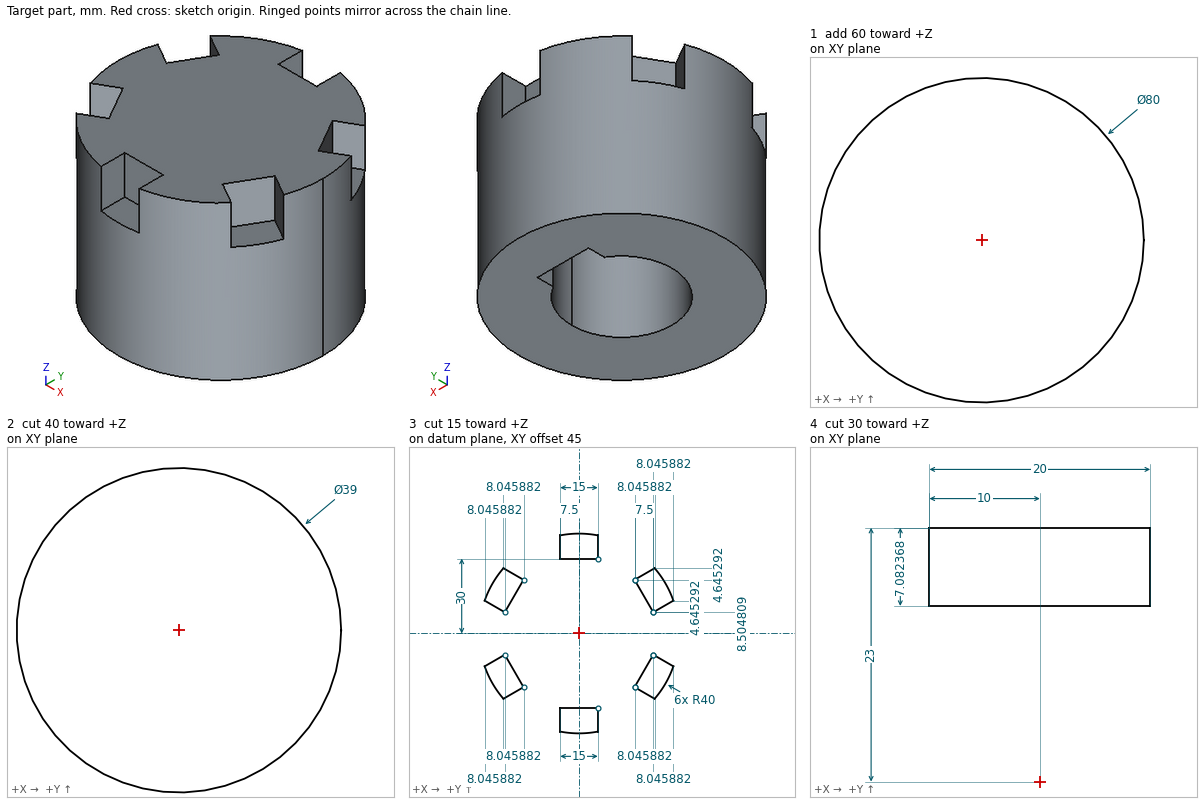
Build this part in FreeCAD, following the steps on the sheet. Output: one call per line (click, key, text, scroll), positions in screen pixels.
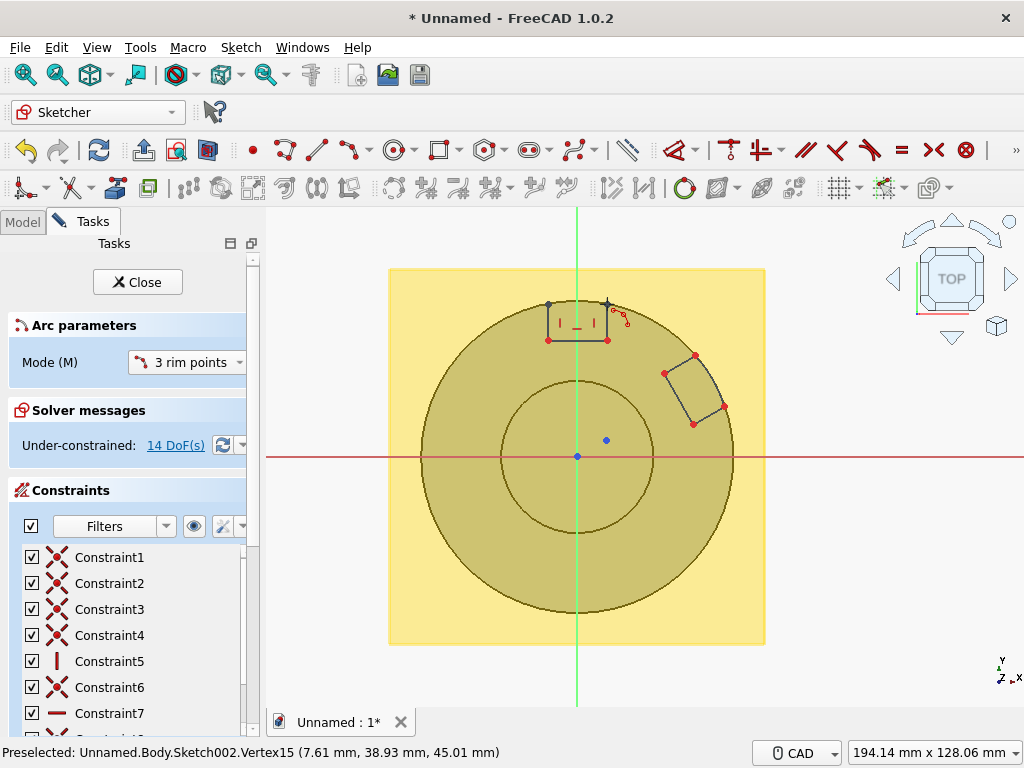
click(607, 305)
click(548, 305)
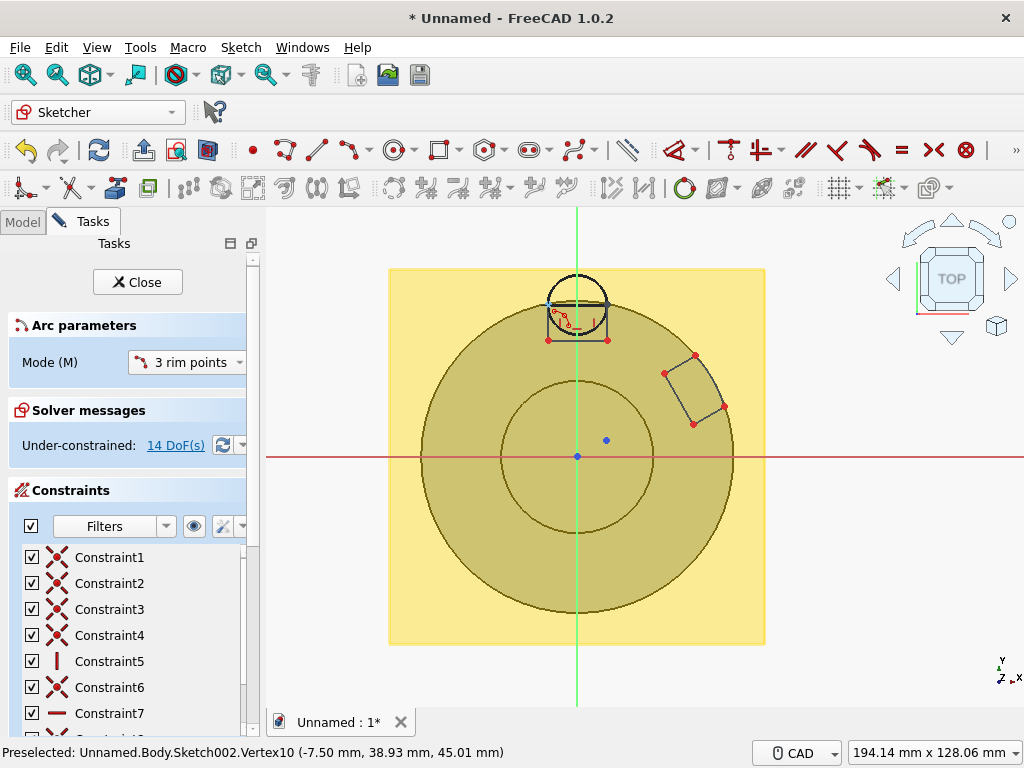
scroll(583, 301, up, 9)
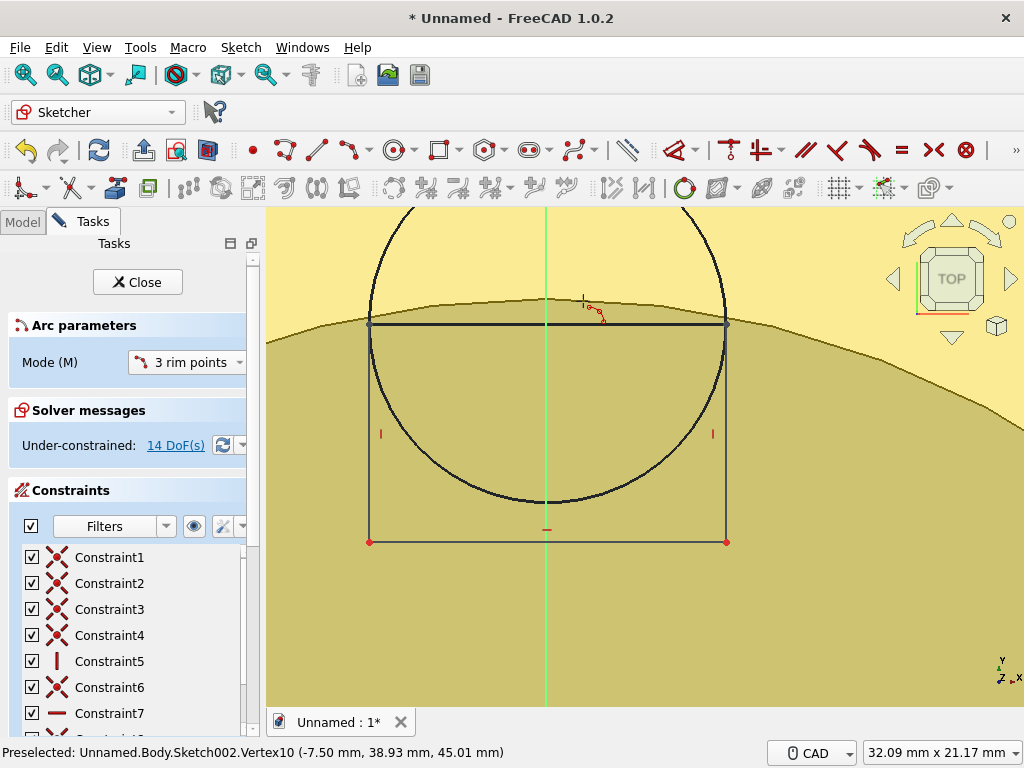
click(582, 300)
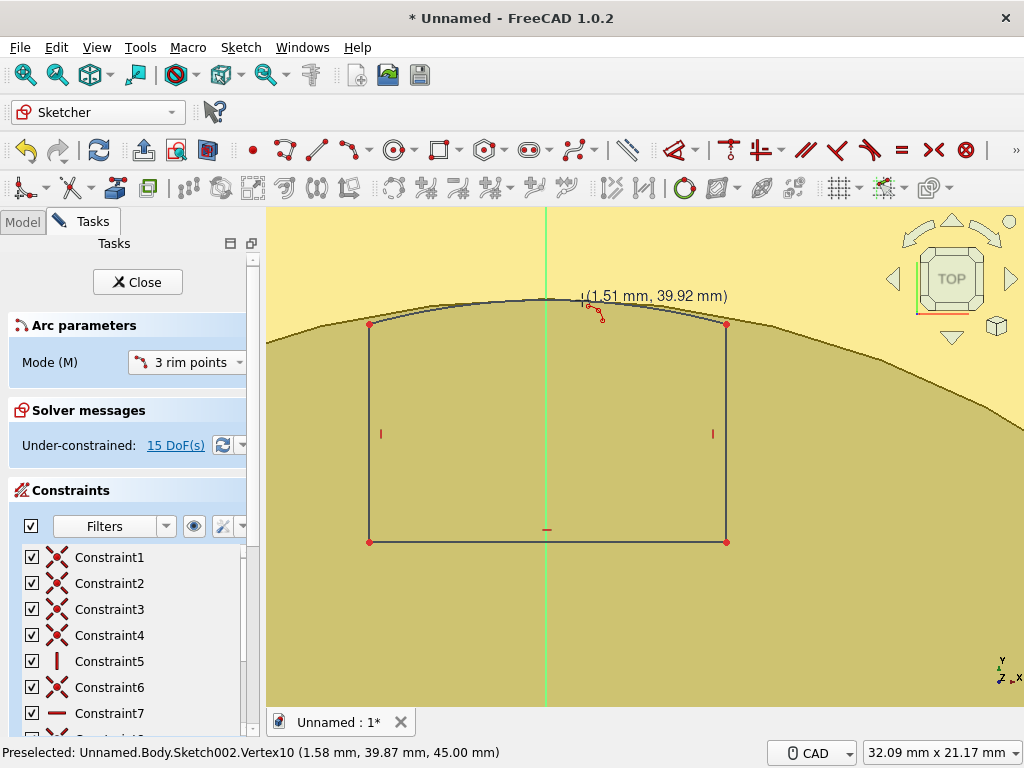
click(286, 150)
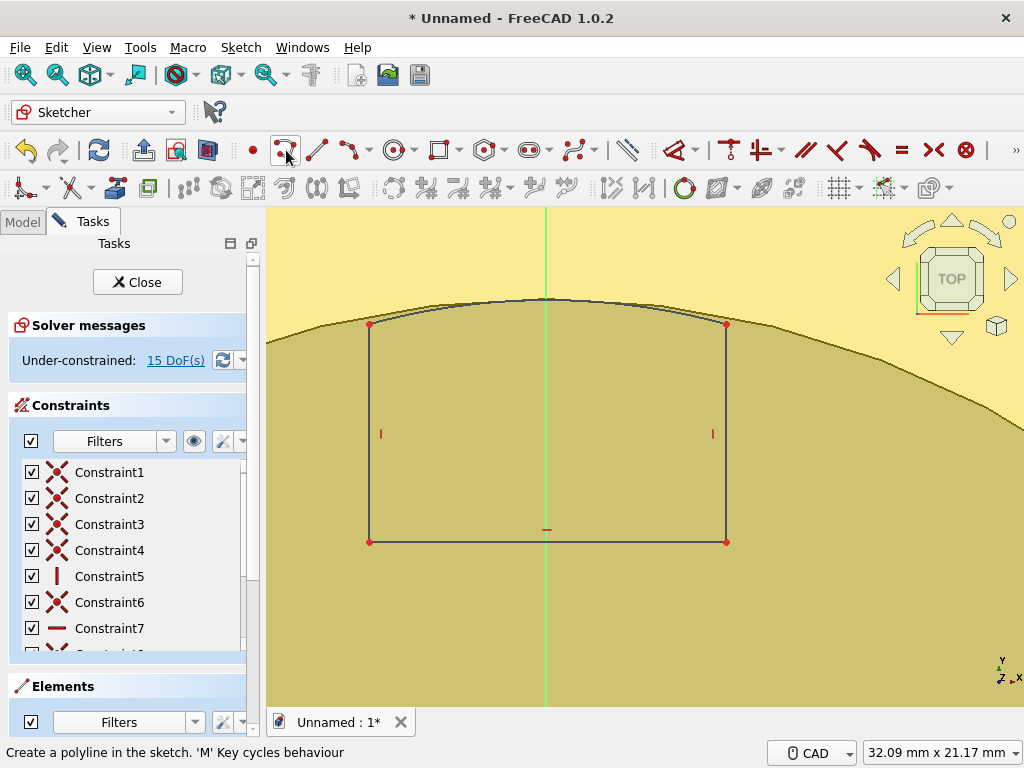
scroll(582, 301, down, 9)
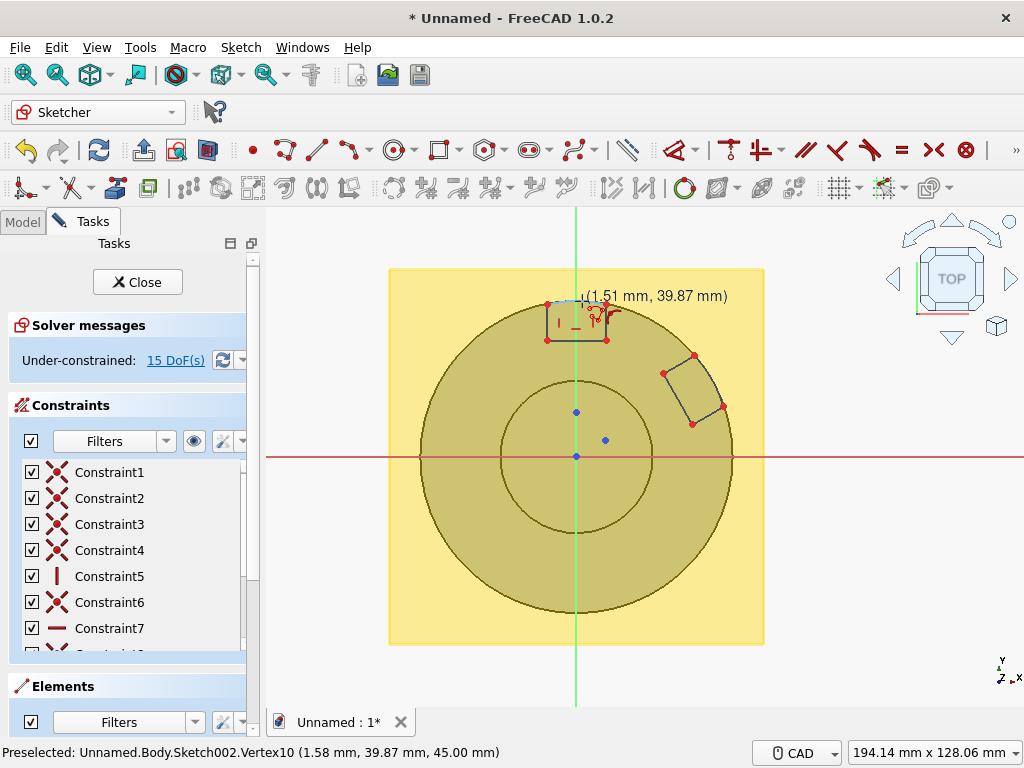
click(724, 508)
click(693, 490)
click(663, 541)
click(695, 559)
right_click(695, 559)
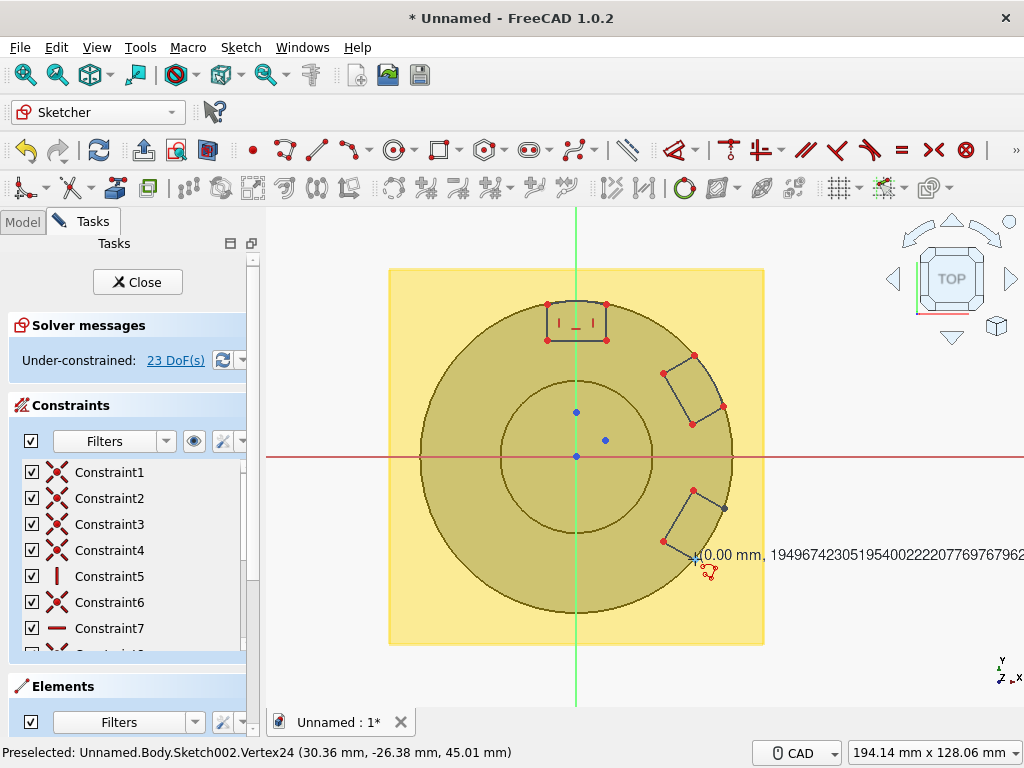
click(350, 150)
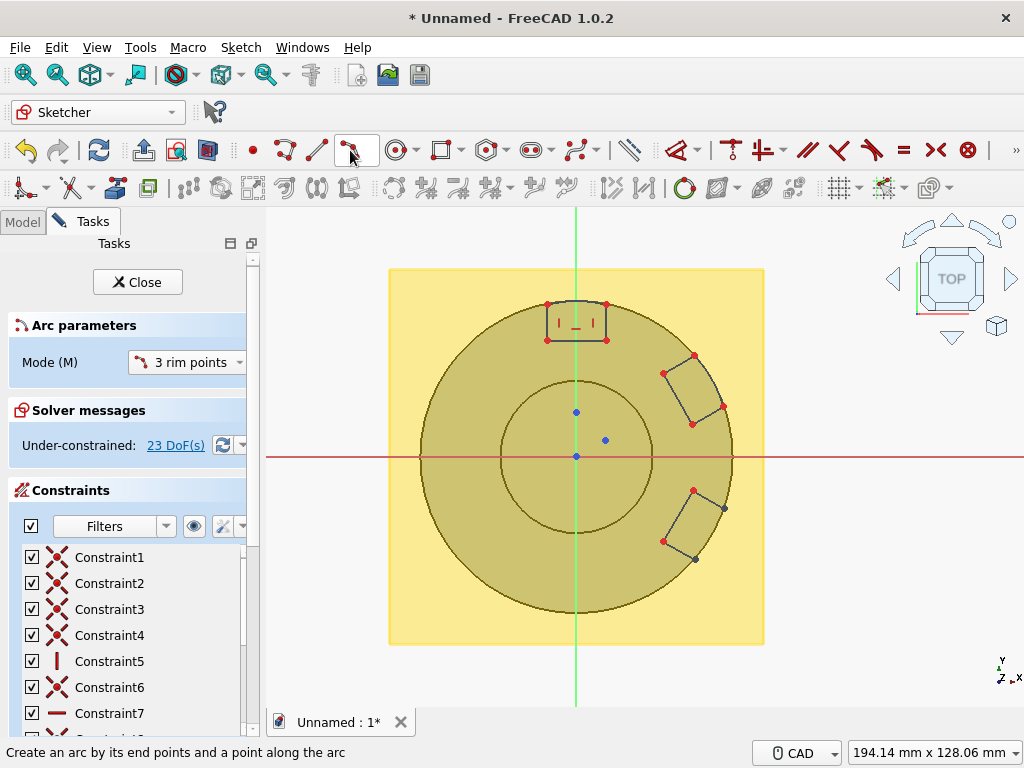
click(695, 560)
click(724, 509)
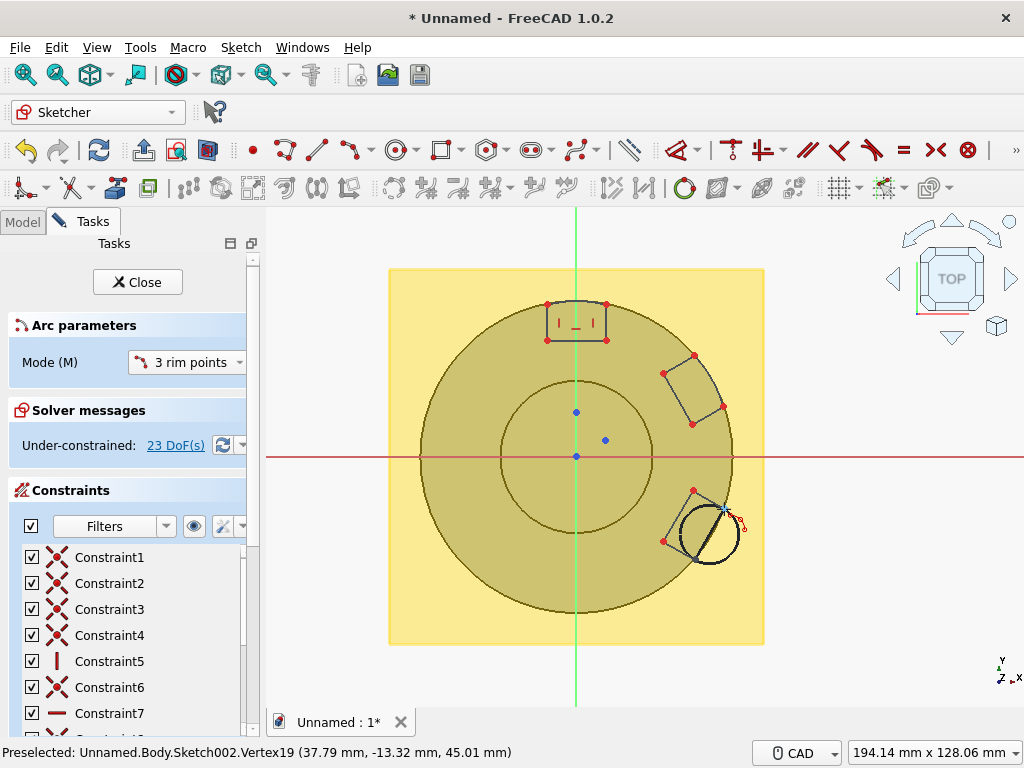
scroll(712, 535, up, 9)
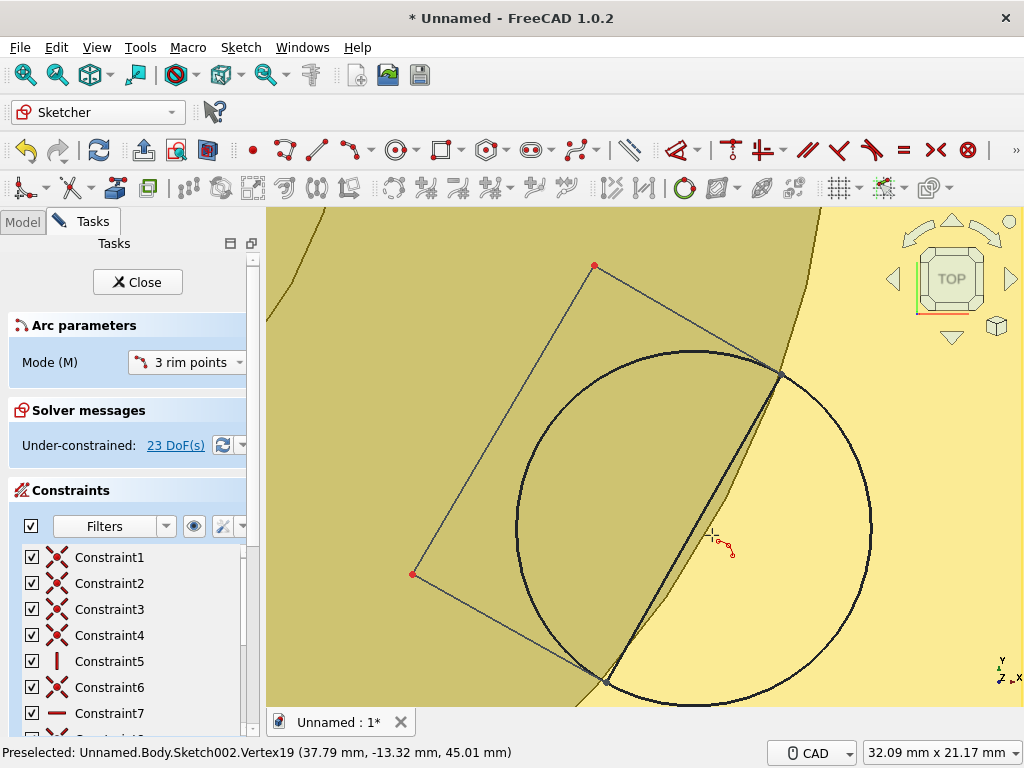
click(707, 532)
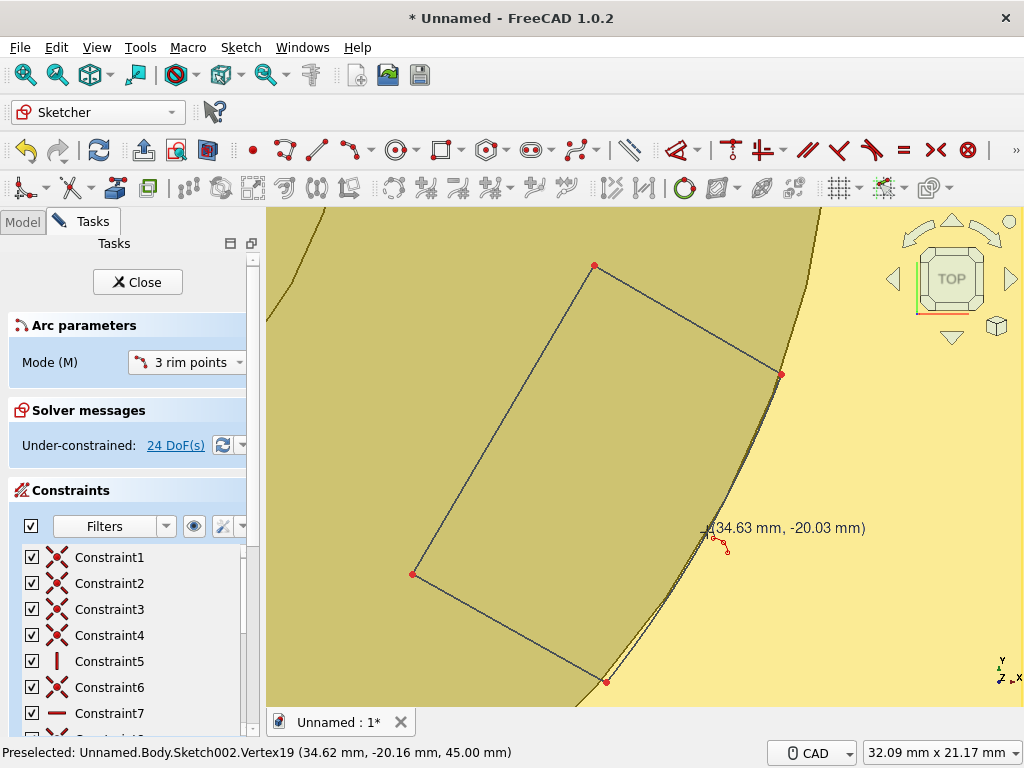
click(286, 150)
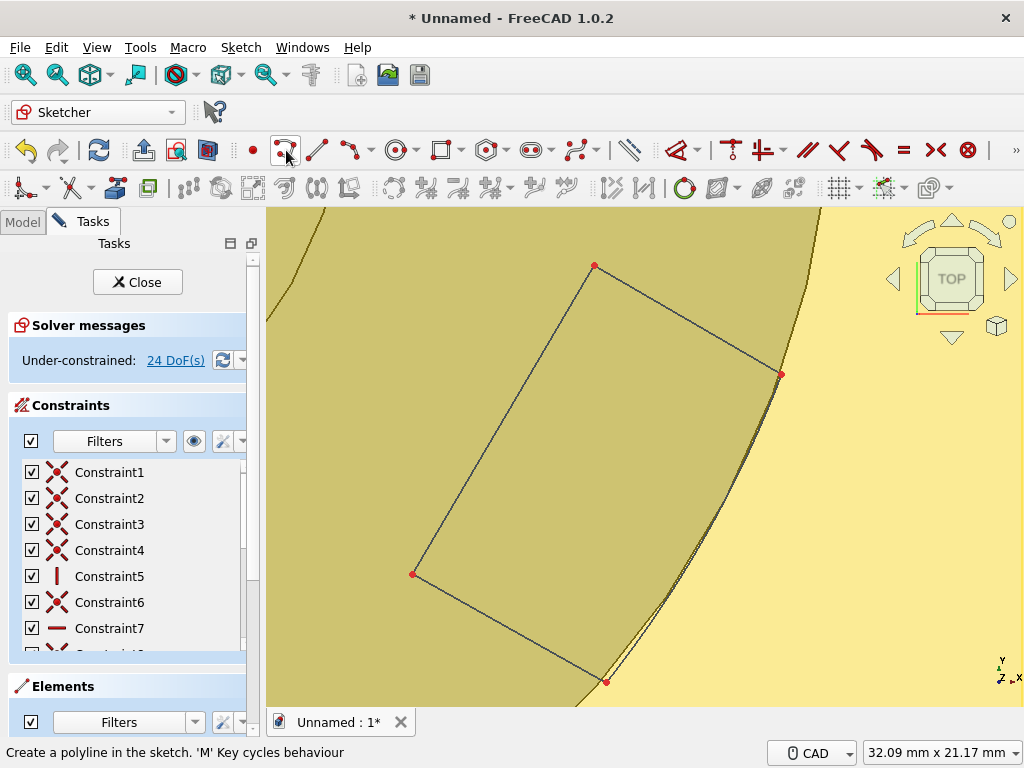
scroll(713, 536, down, 9)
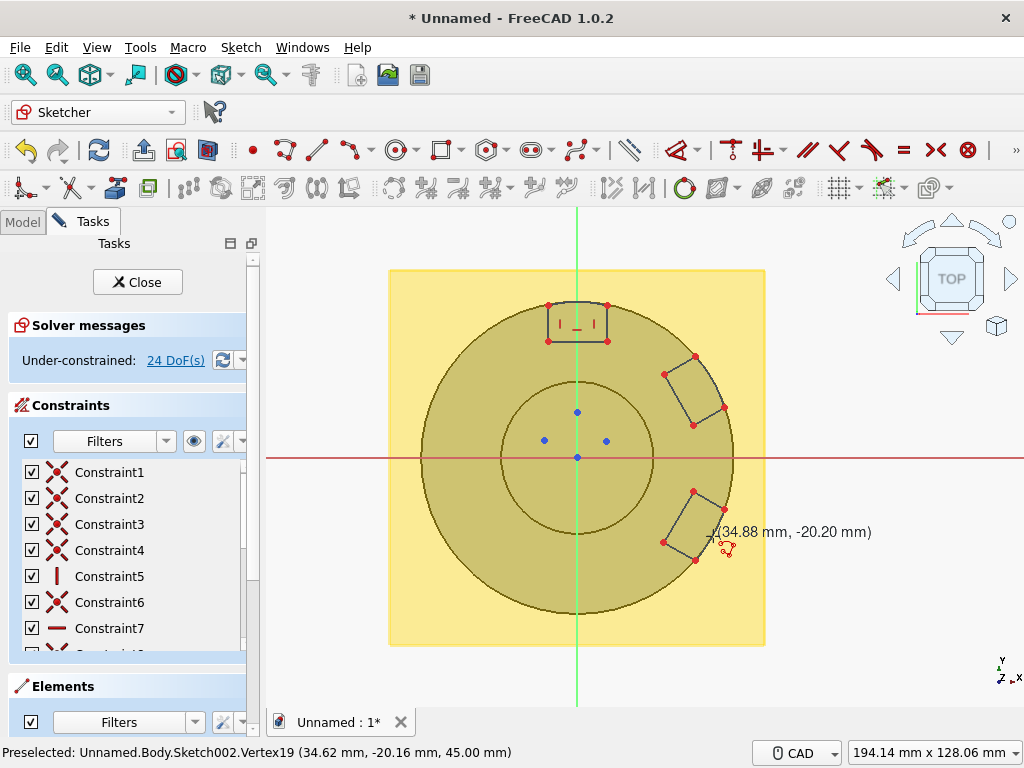
click(607, 611)
click(607, 575)
click(548, 575)
click(548, 611)
right_click(548, 611)